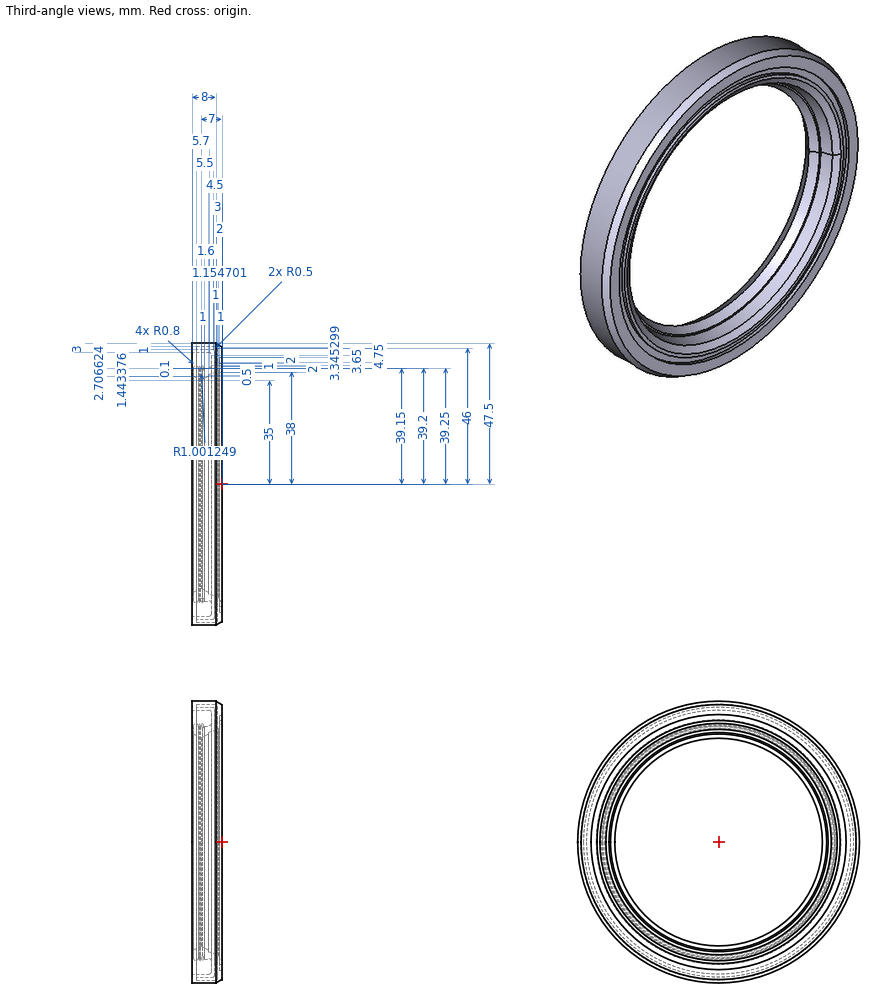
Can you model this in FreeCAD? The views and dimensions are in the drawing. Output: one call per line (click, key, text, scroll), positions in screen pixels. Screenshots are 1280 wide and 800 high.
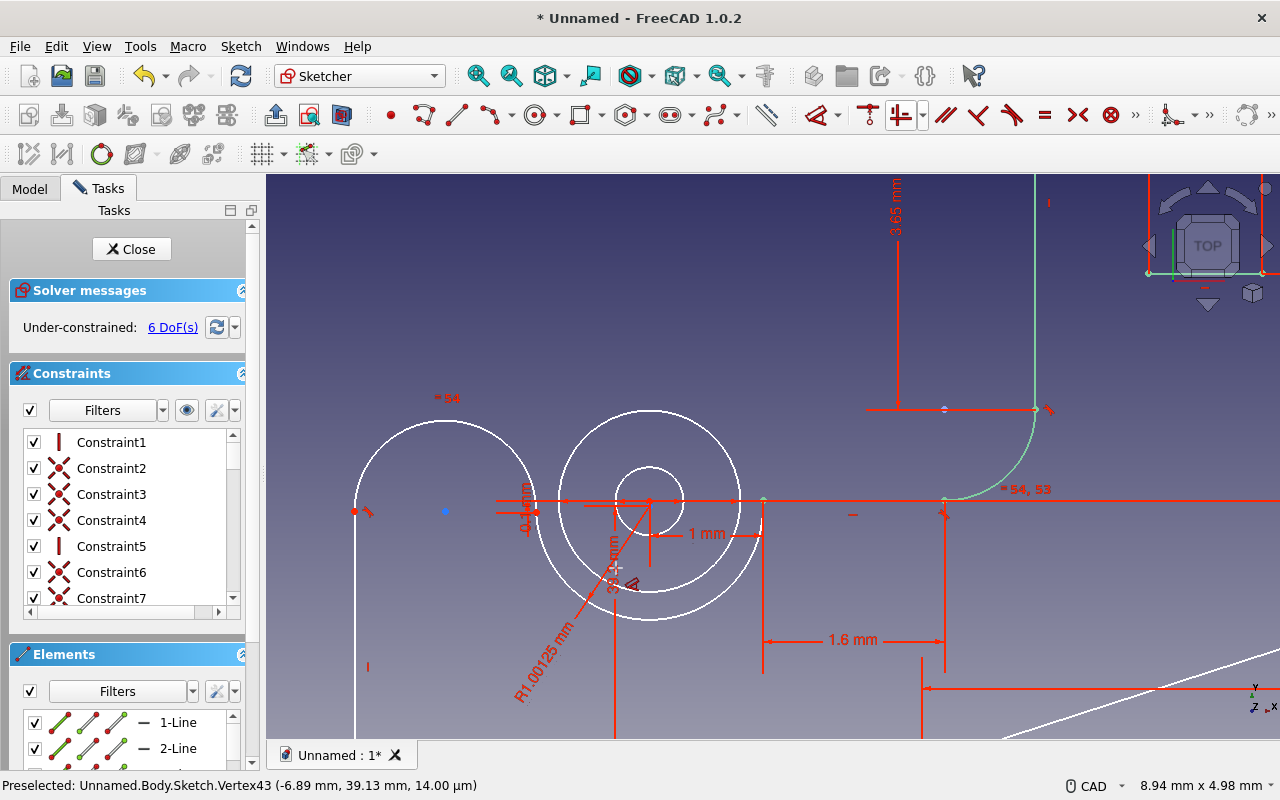
scroll(650, 501, up, 5)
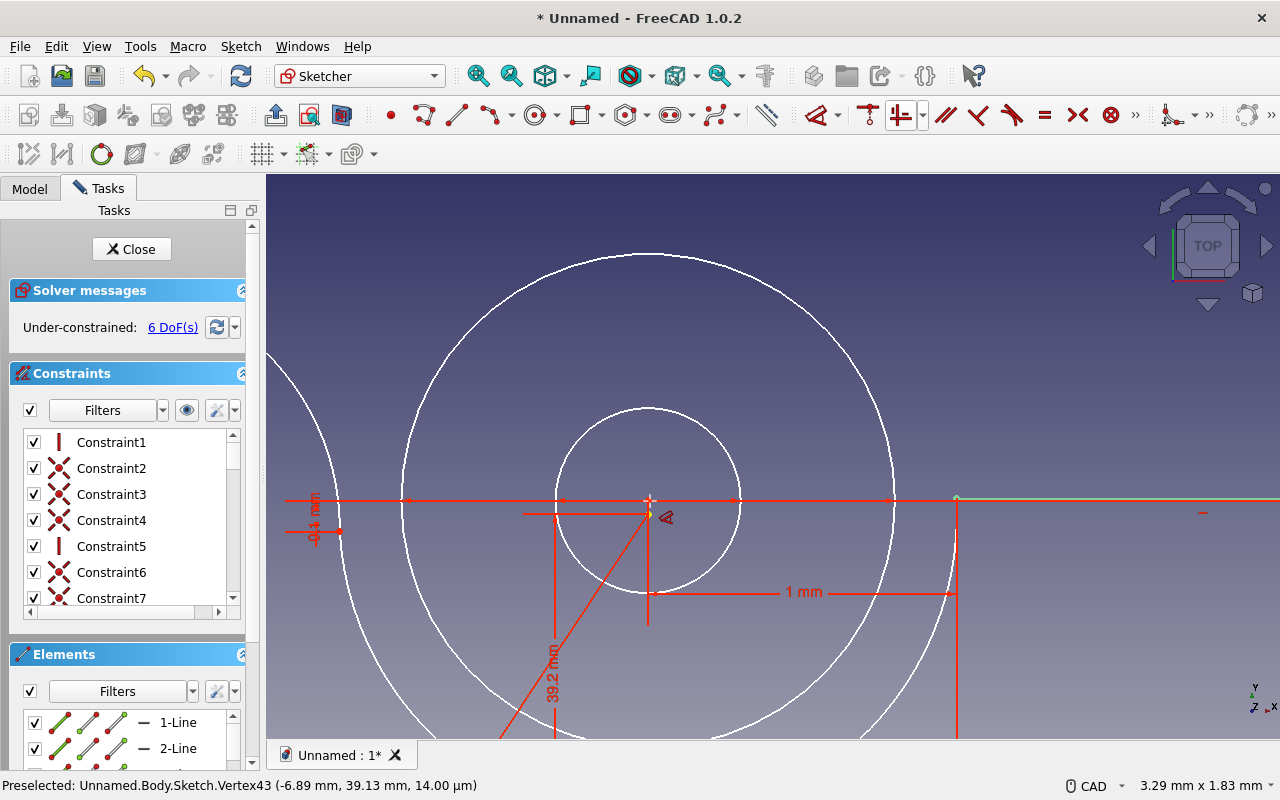
click(648, 501)
click(614, 606)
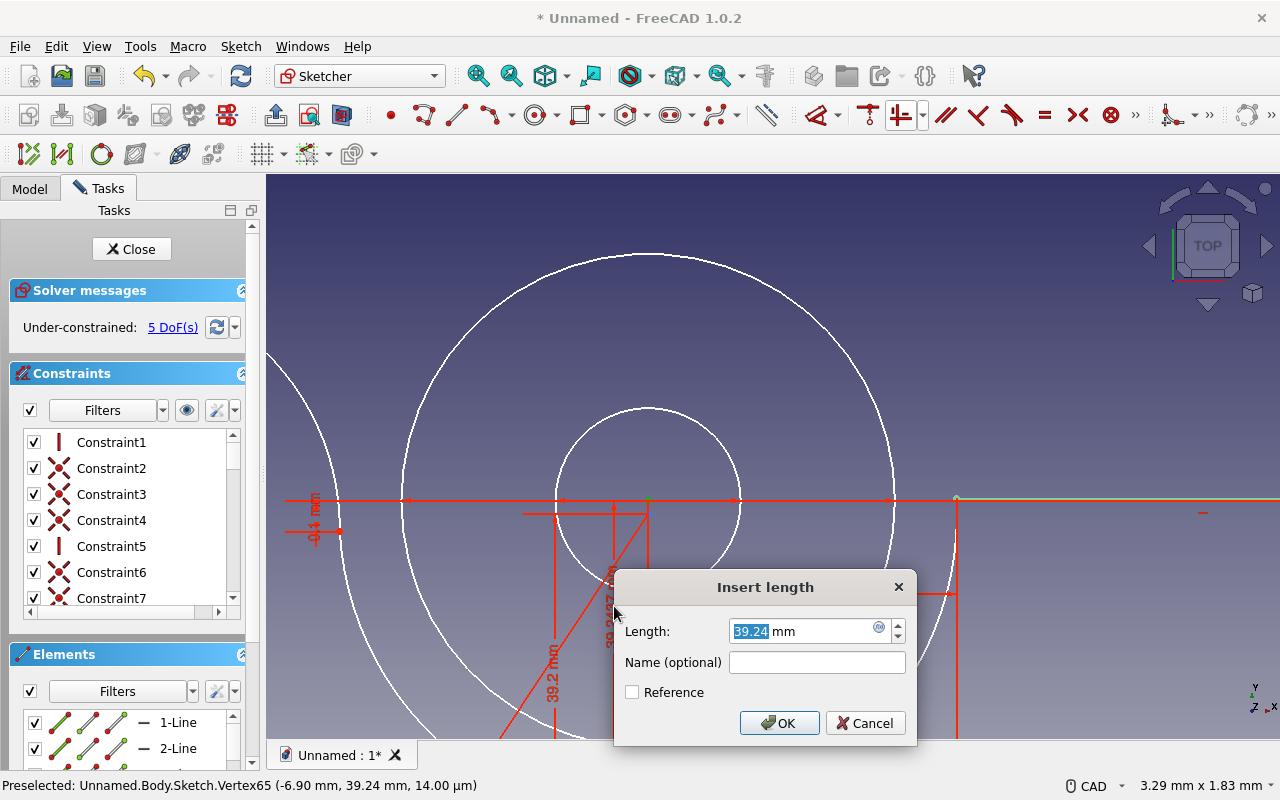
text(39.25)
key(Return)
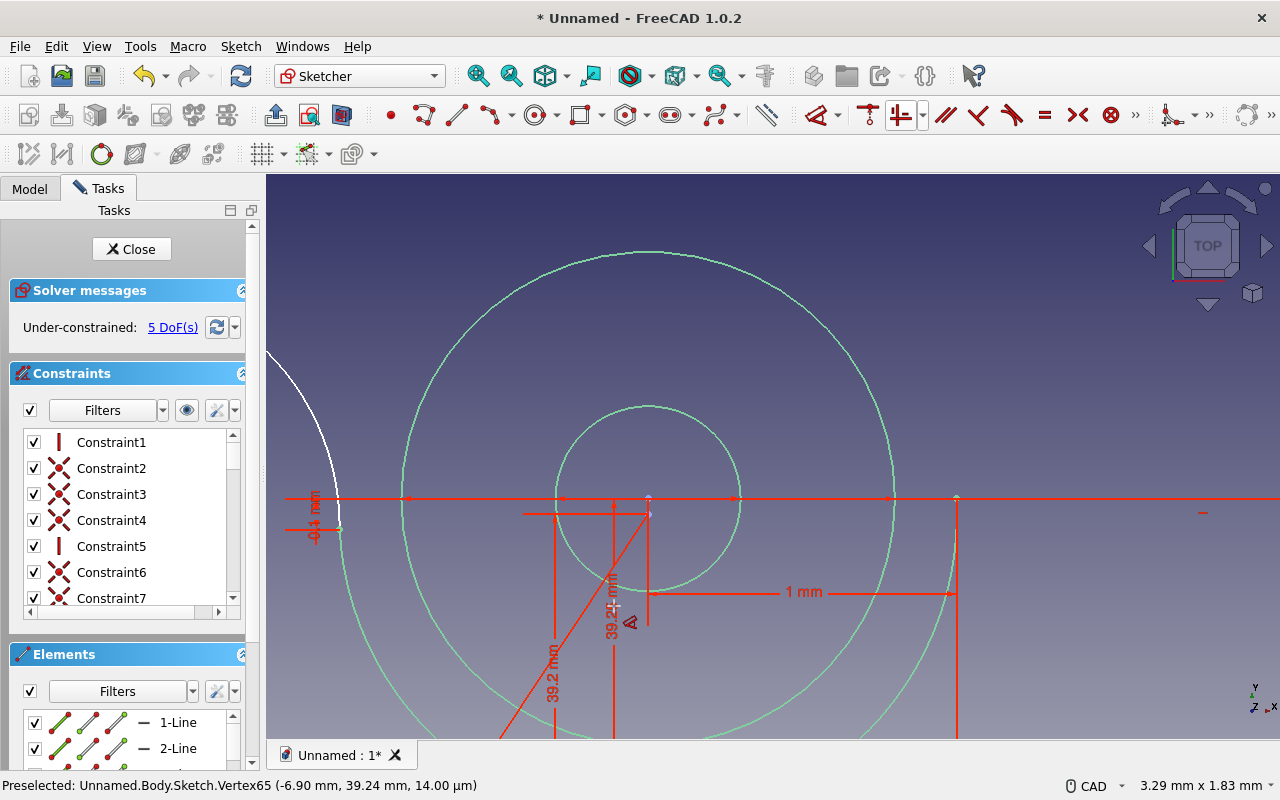
scroll(652, 514, down, 12)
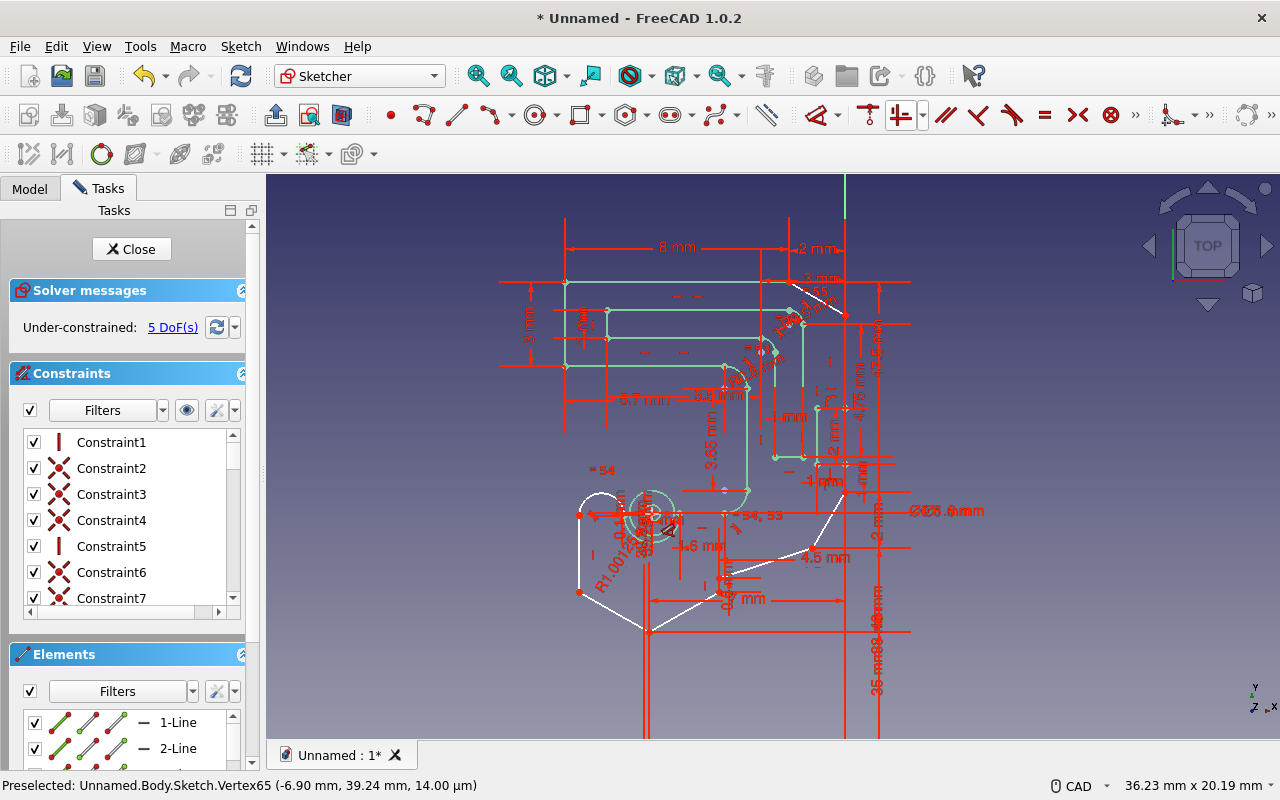
click(579, 516)
click(545, 613)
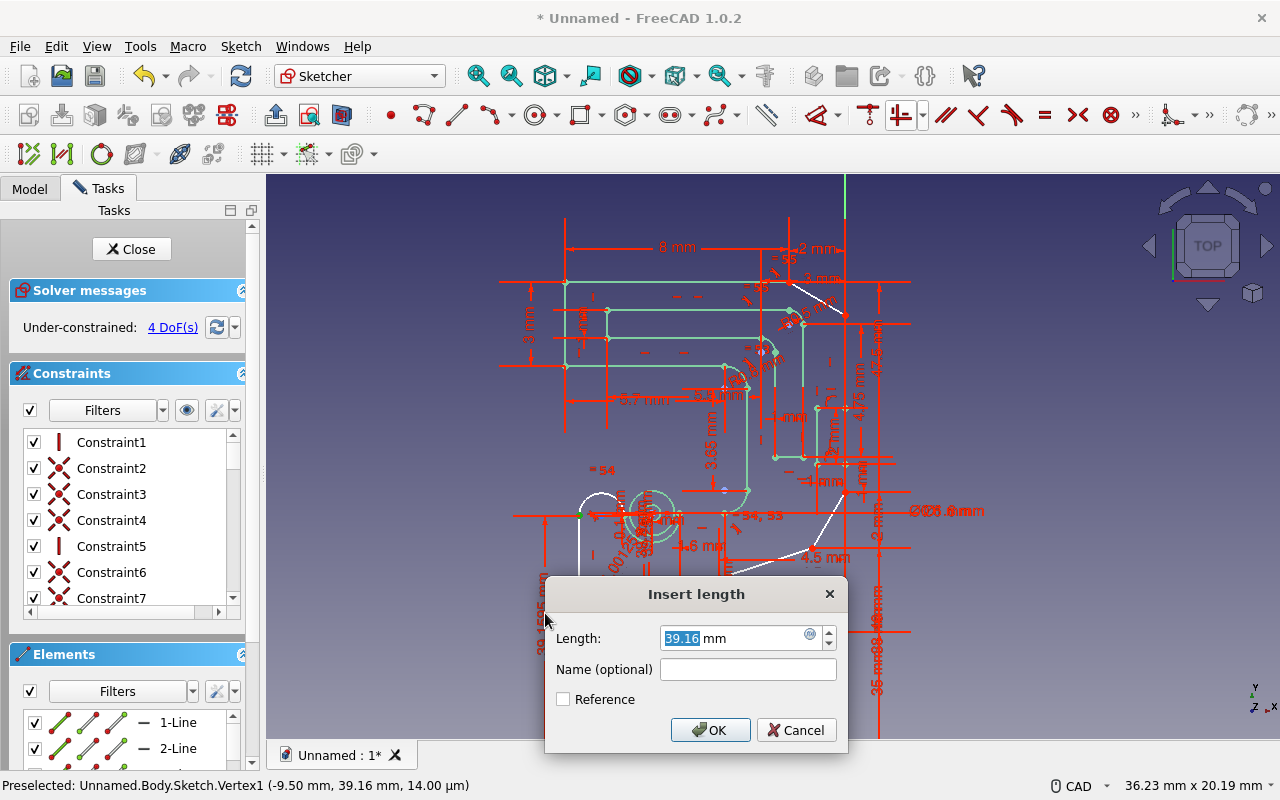
text(39.15)
key(Return)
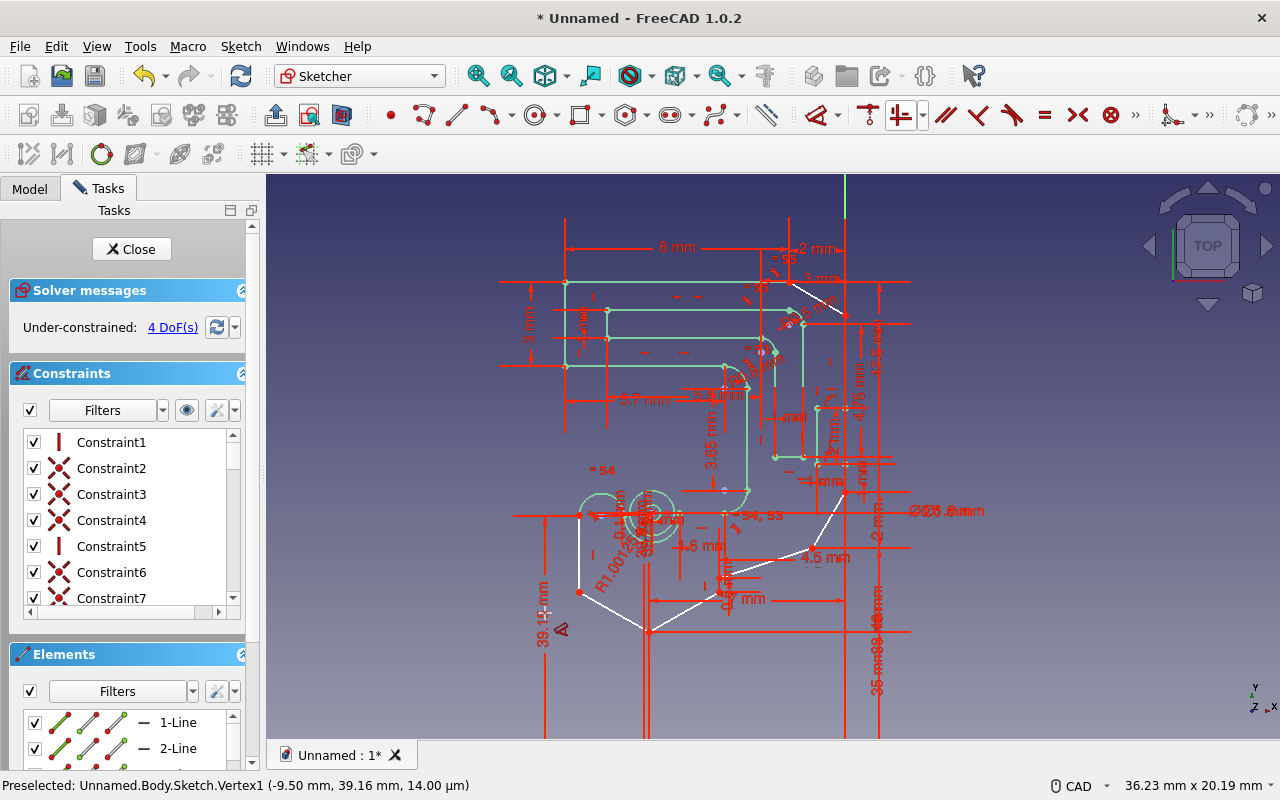
click(579, 539)
click(545, 554)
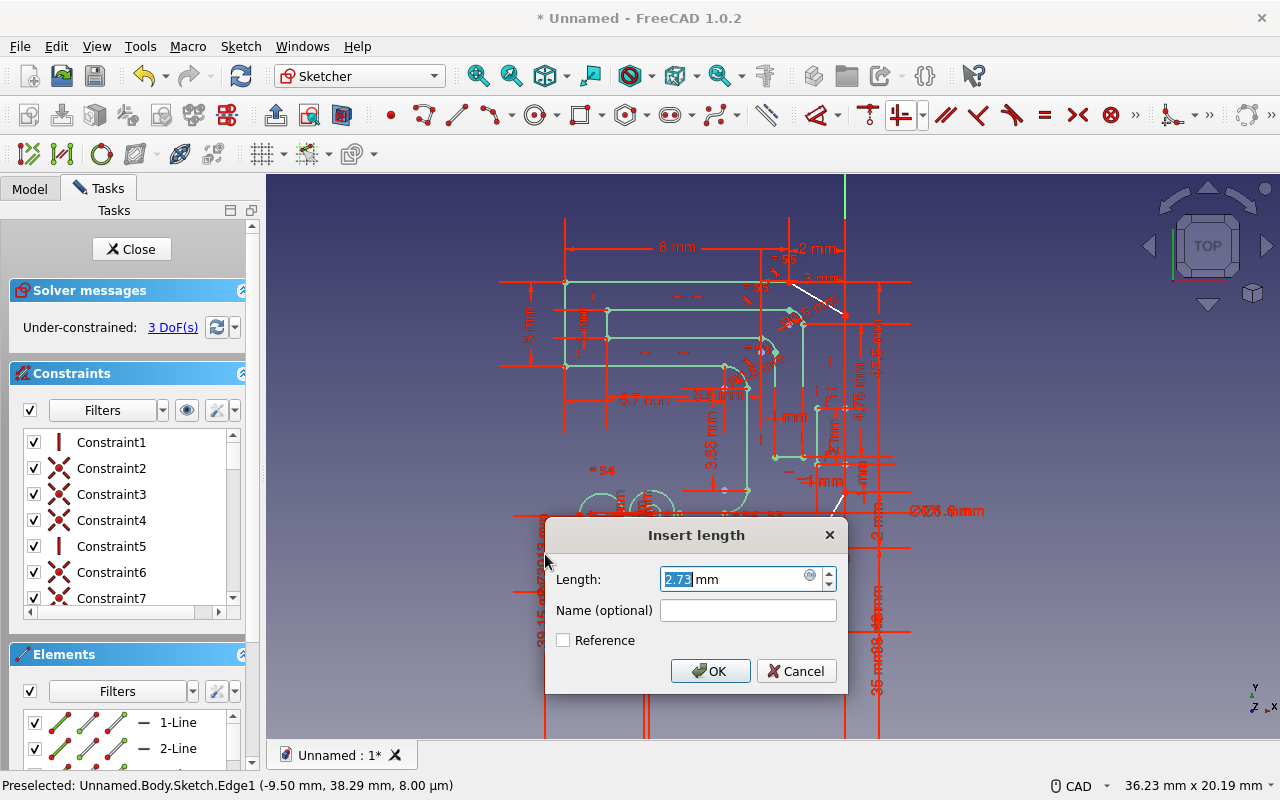
text(2.706624)
key(Return)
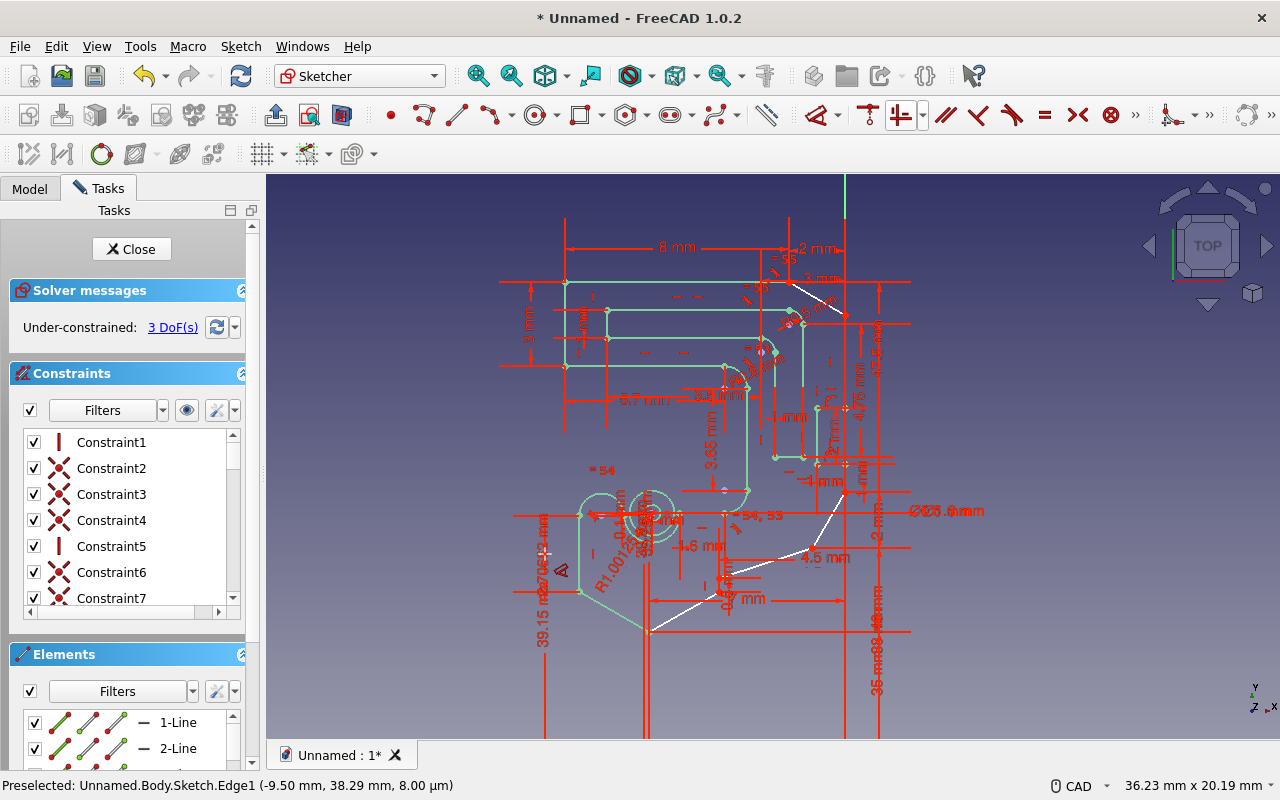
click(845, 380)
click(787, 340)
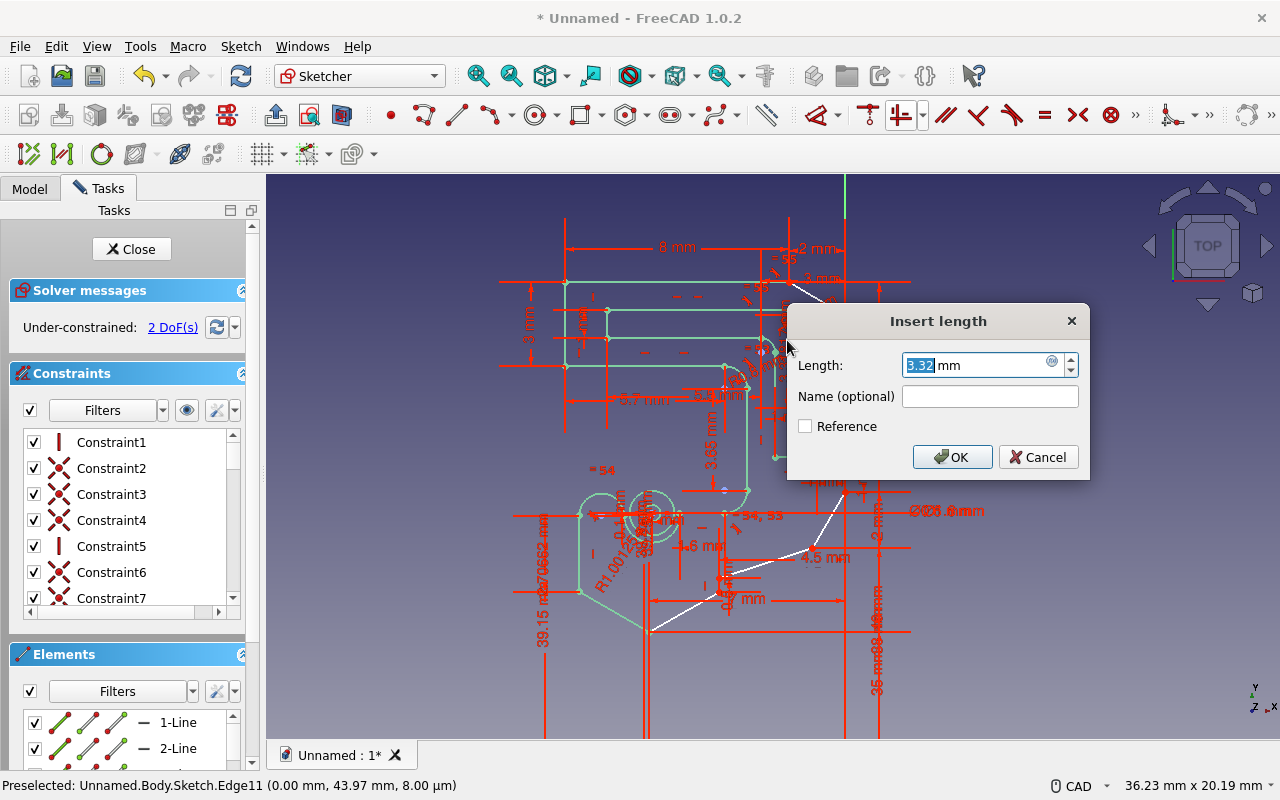
text(3.345299)
key(Return)